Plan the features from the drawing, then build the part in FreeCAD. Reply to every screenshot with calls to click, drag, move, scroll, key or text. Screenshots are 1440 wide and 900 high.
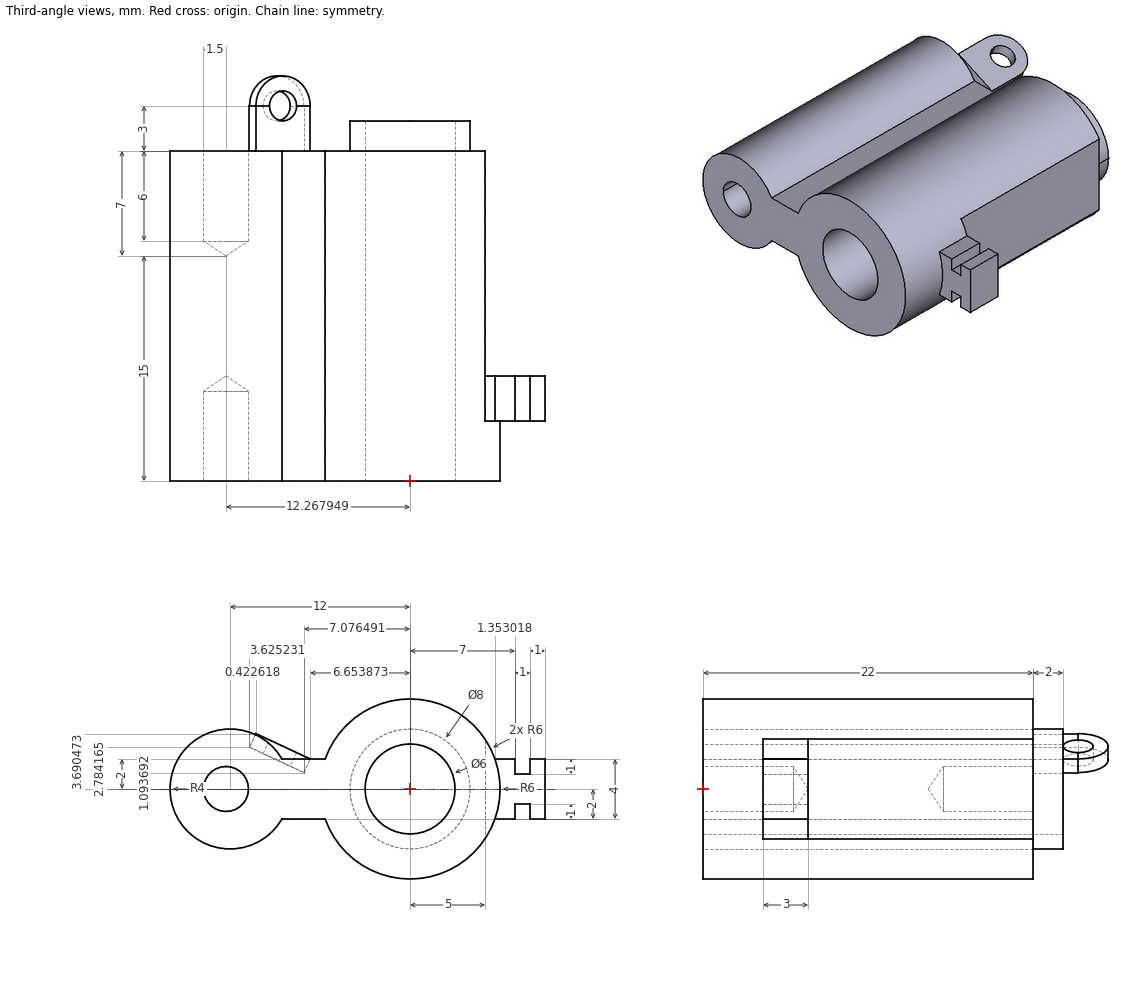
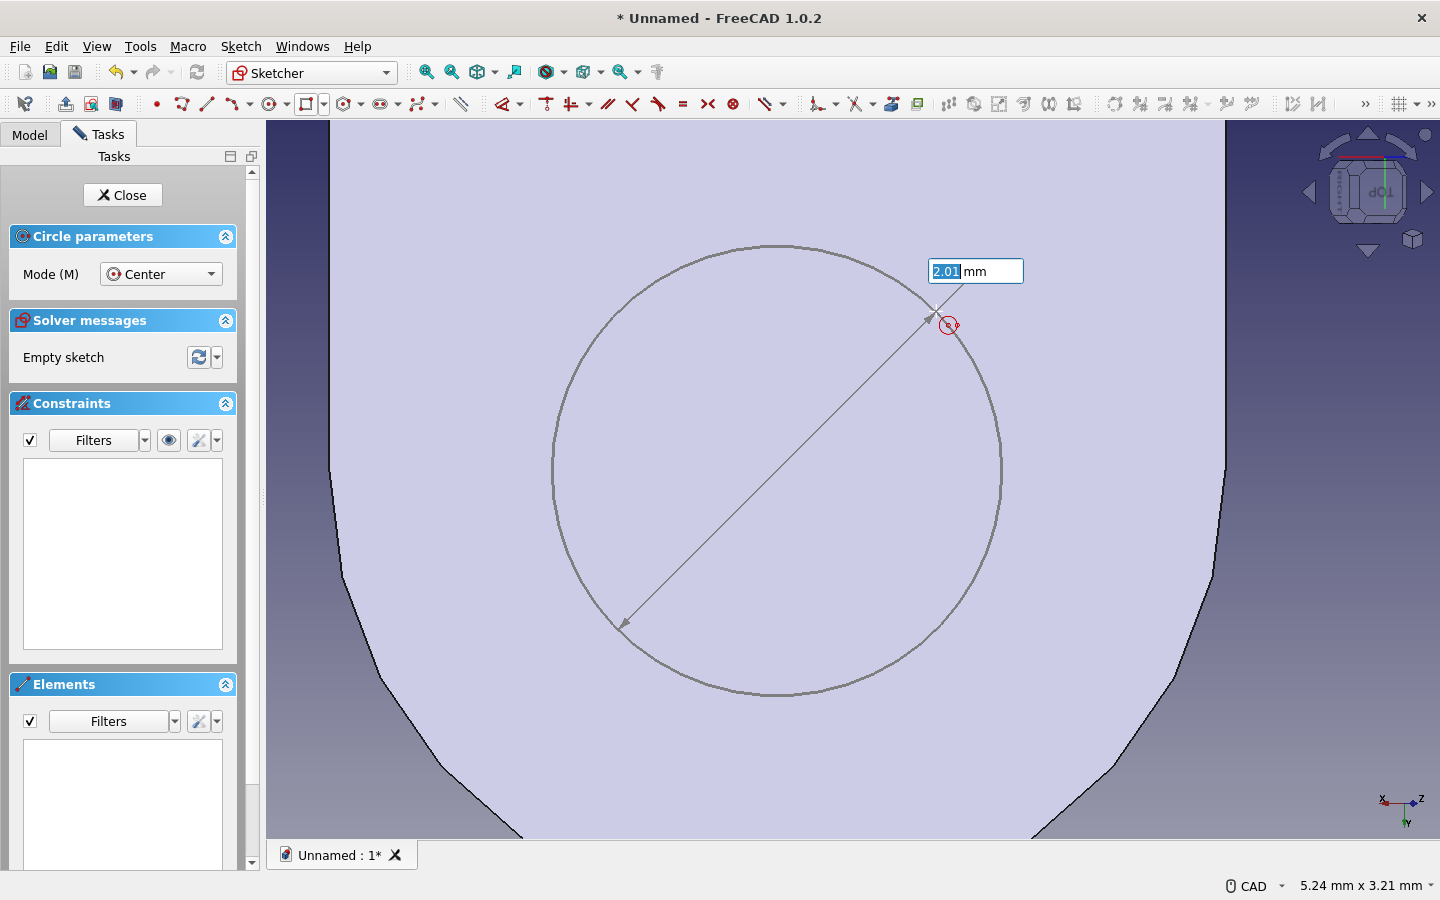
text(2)
key(Return)
key(Escape)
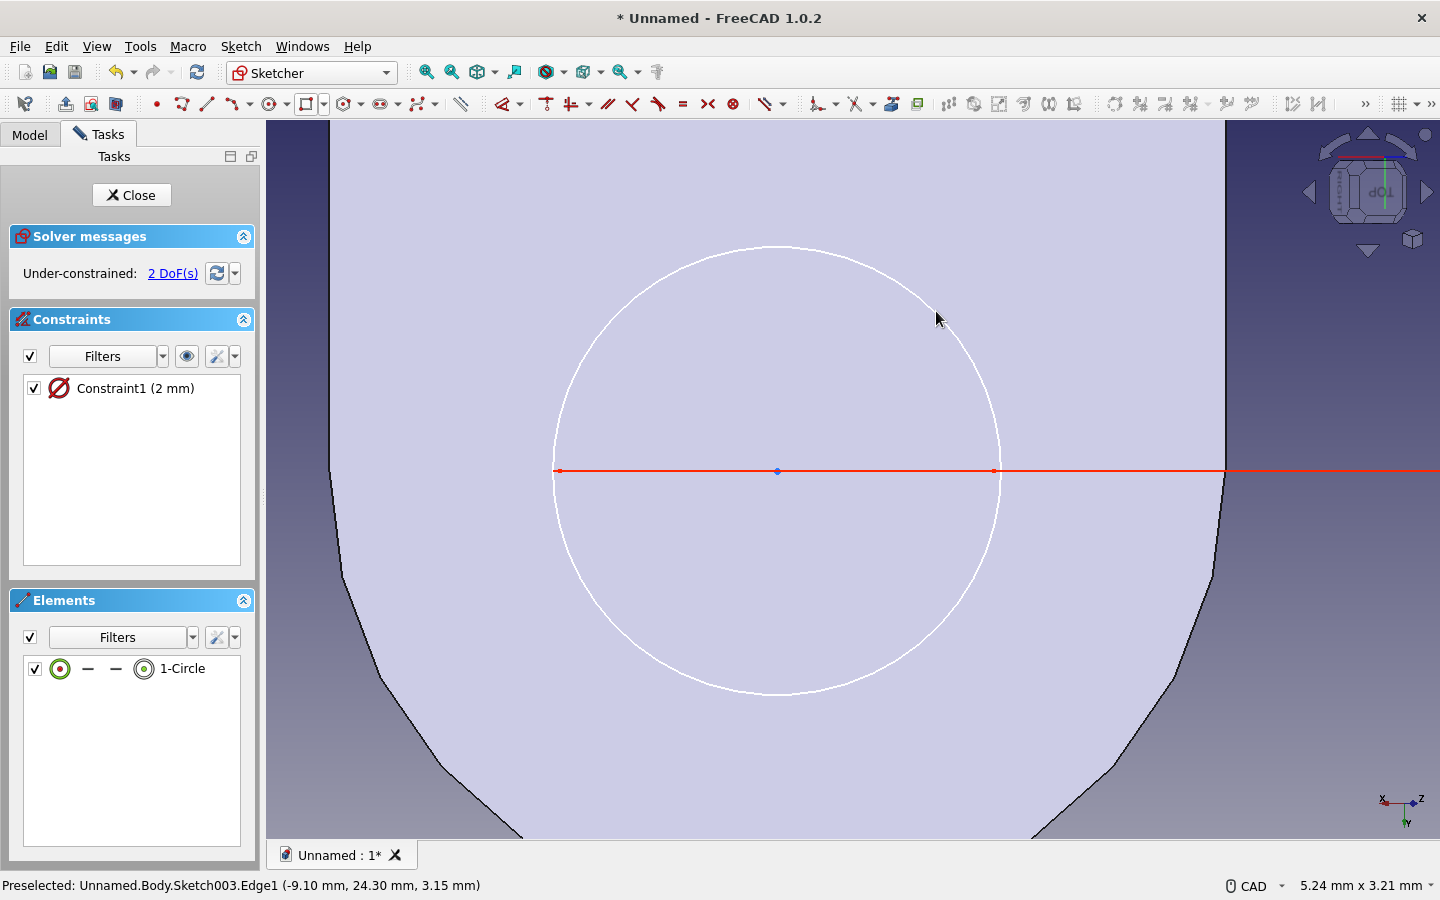
click(502, 104)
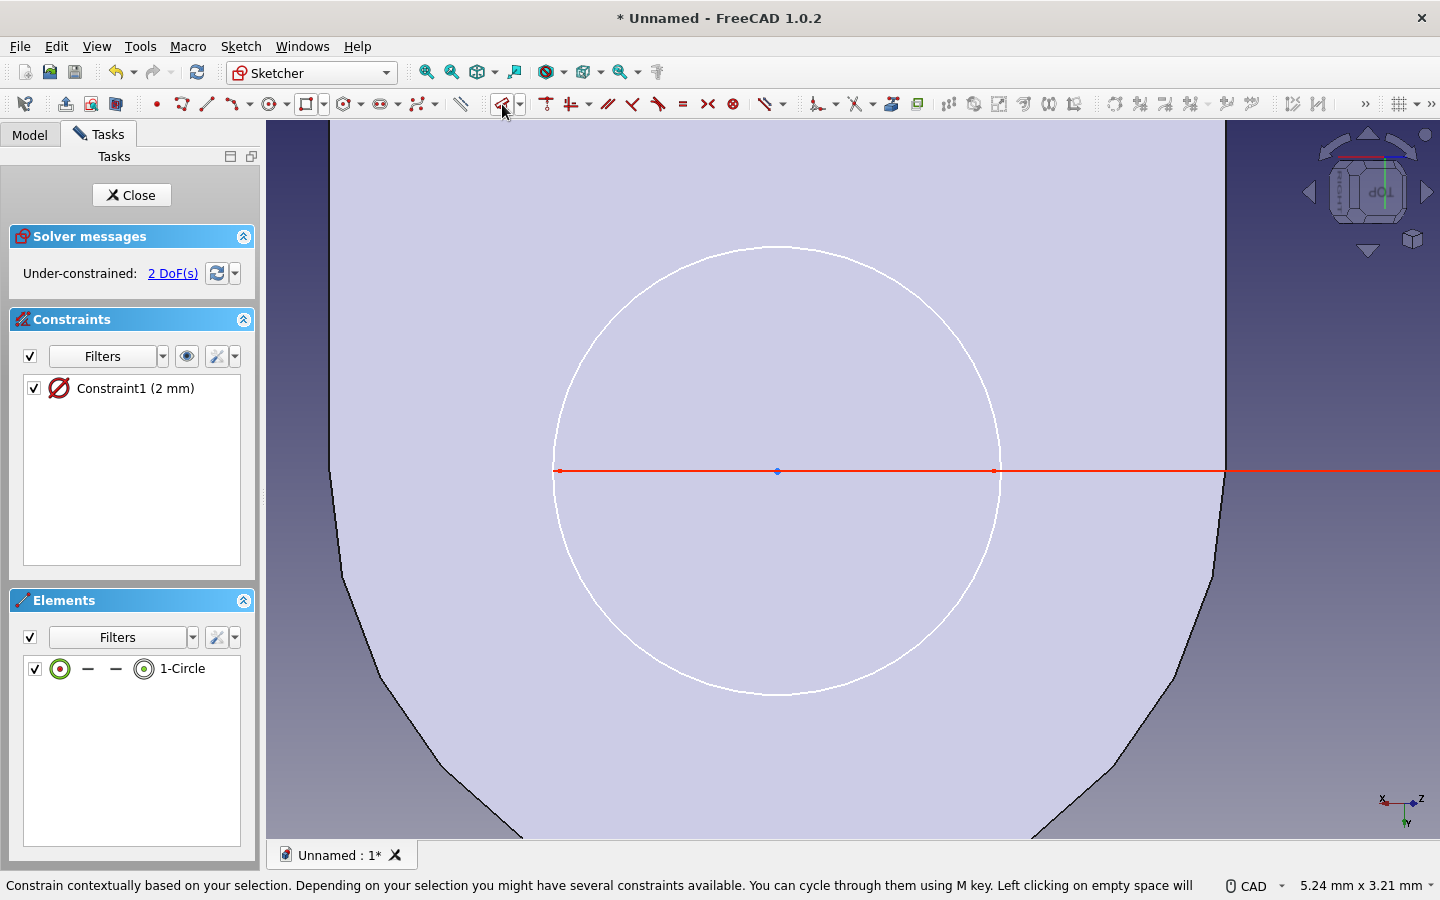
click(777, 471)
click(811, 310)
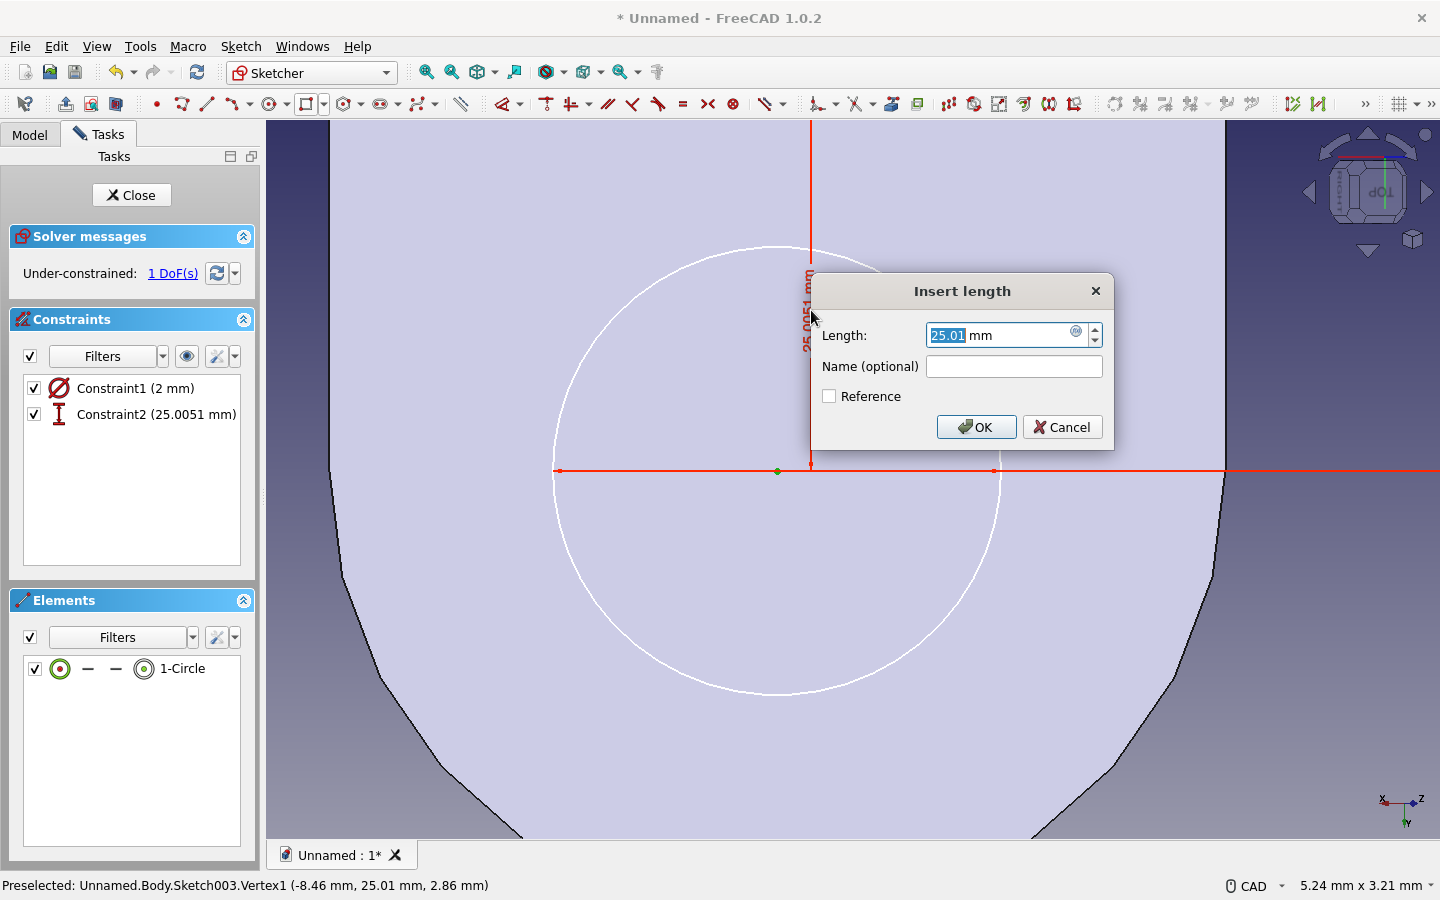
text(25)
key(Return)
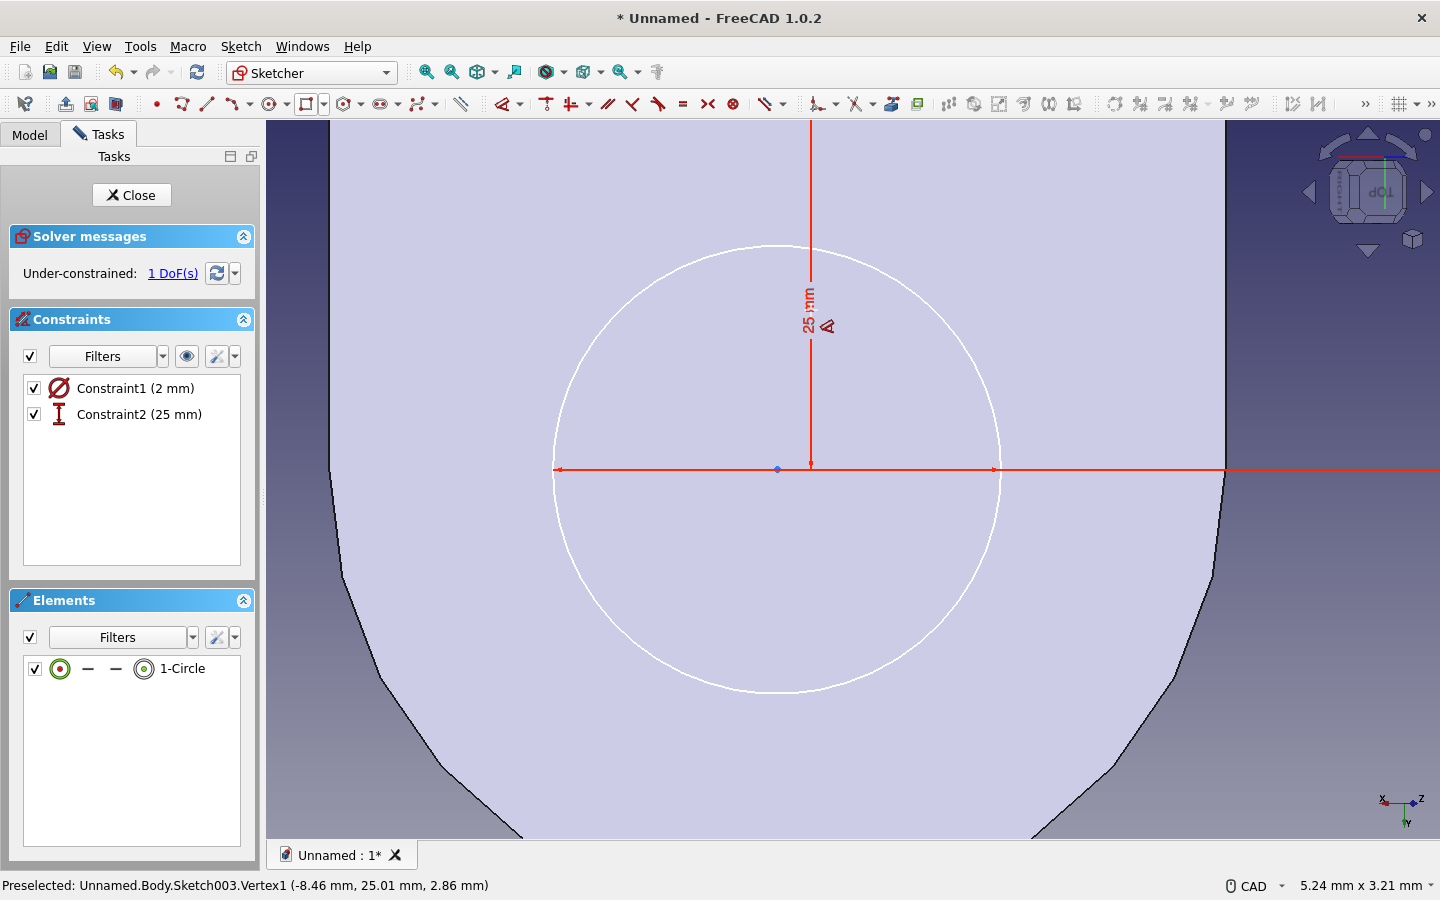
click(777, 470)
click(536, 504)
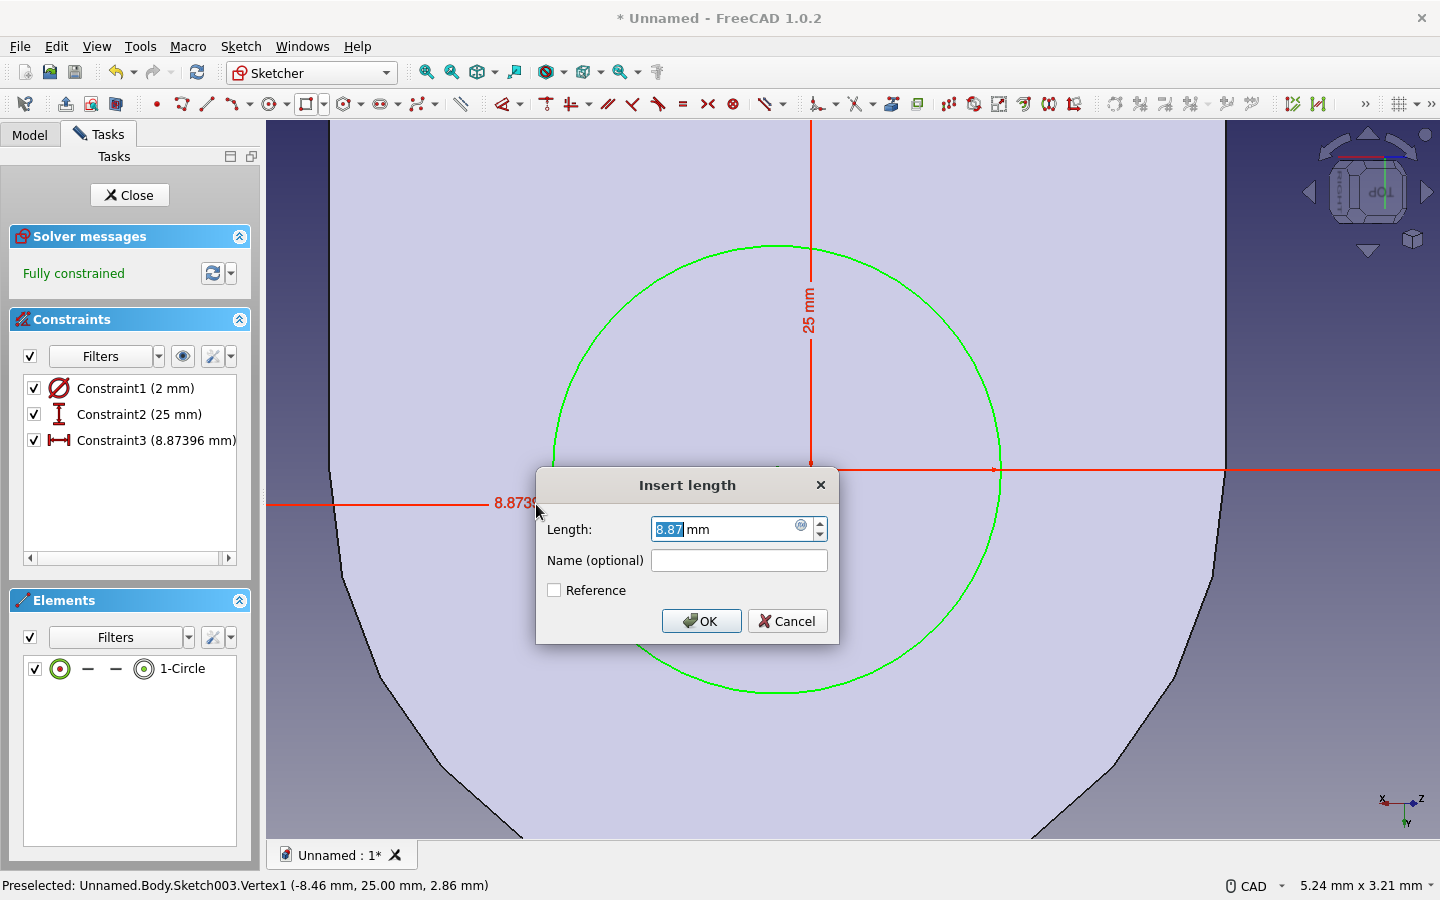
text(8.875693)
key(Return)
key(Escape)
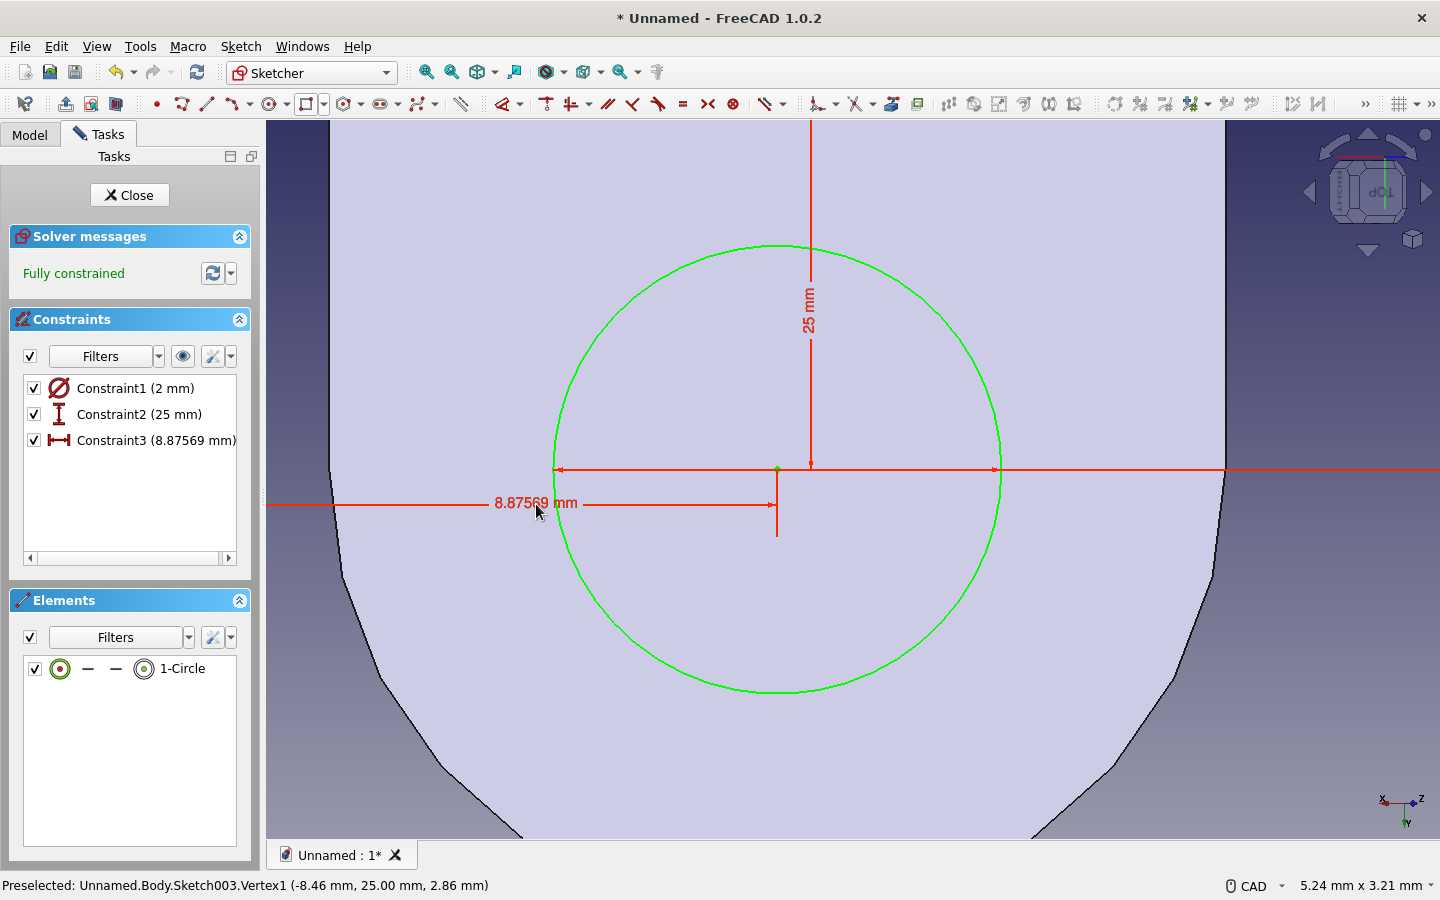
click(130, 195)